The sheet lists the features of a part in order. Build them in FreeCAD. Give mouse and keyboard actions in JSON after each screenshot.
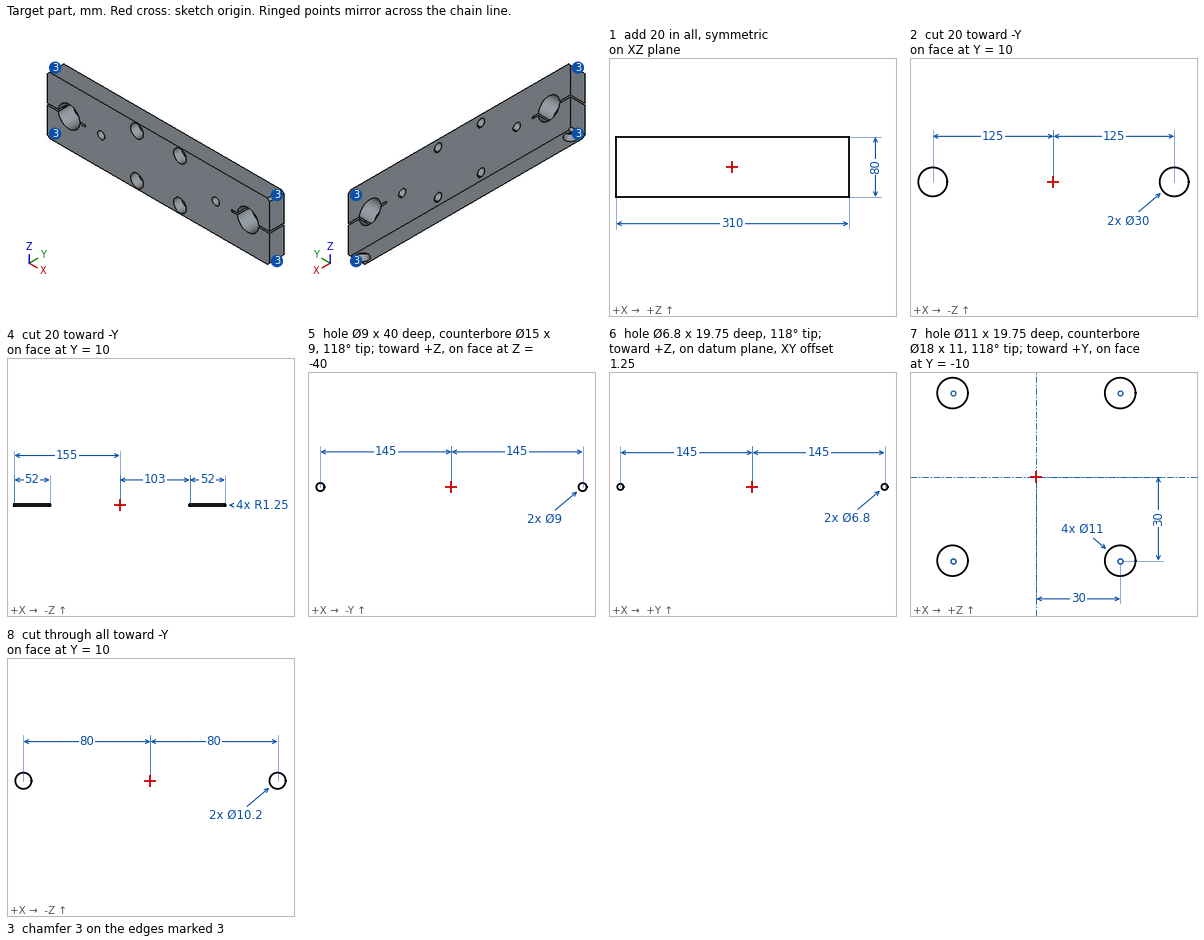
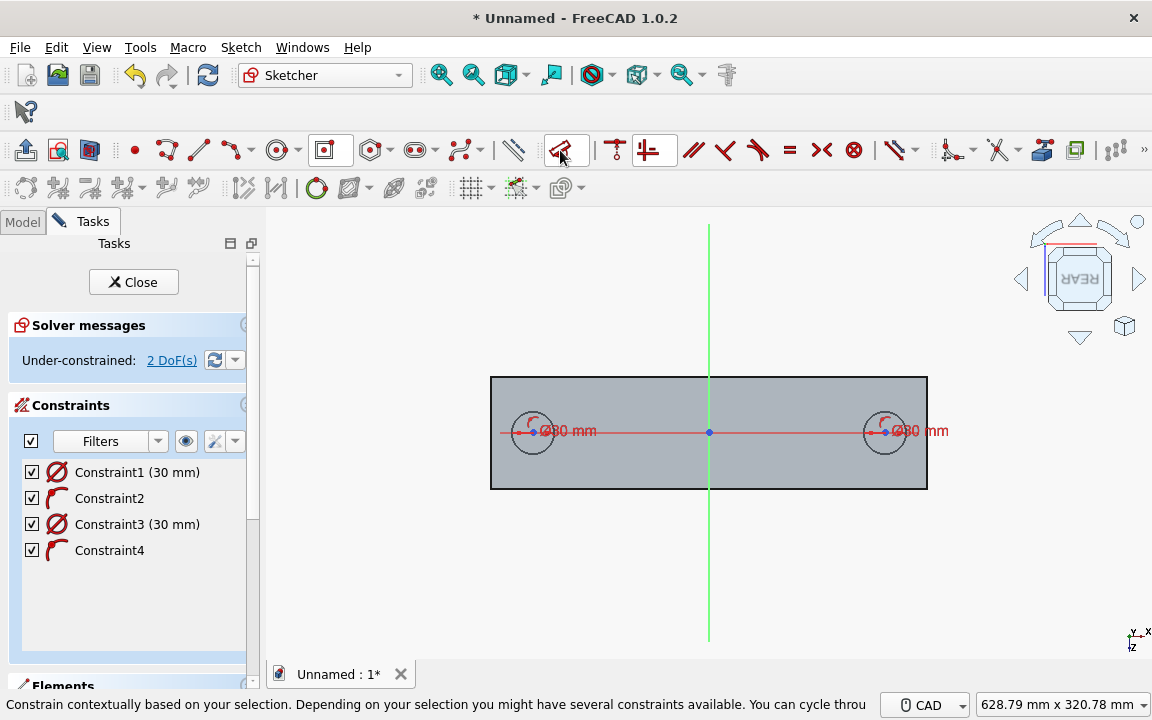
{"action": "left_click", "coordinate": [885, 433]}
{"action": "left_click", "coordinate": [797, 467]}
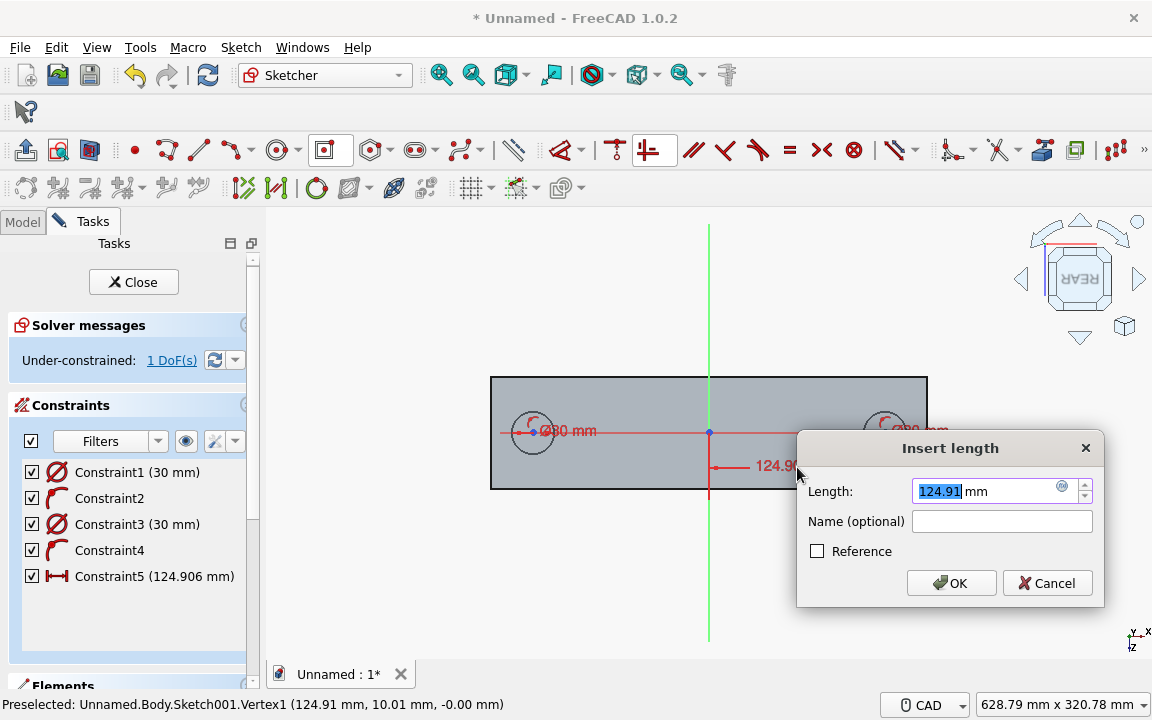
{"action": "type", "text": "125"}
{"action": "key", "text": "Return"}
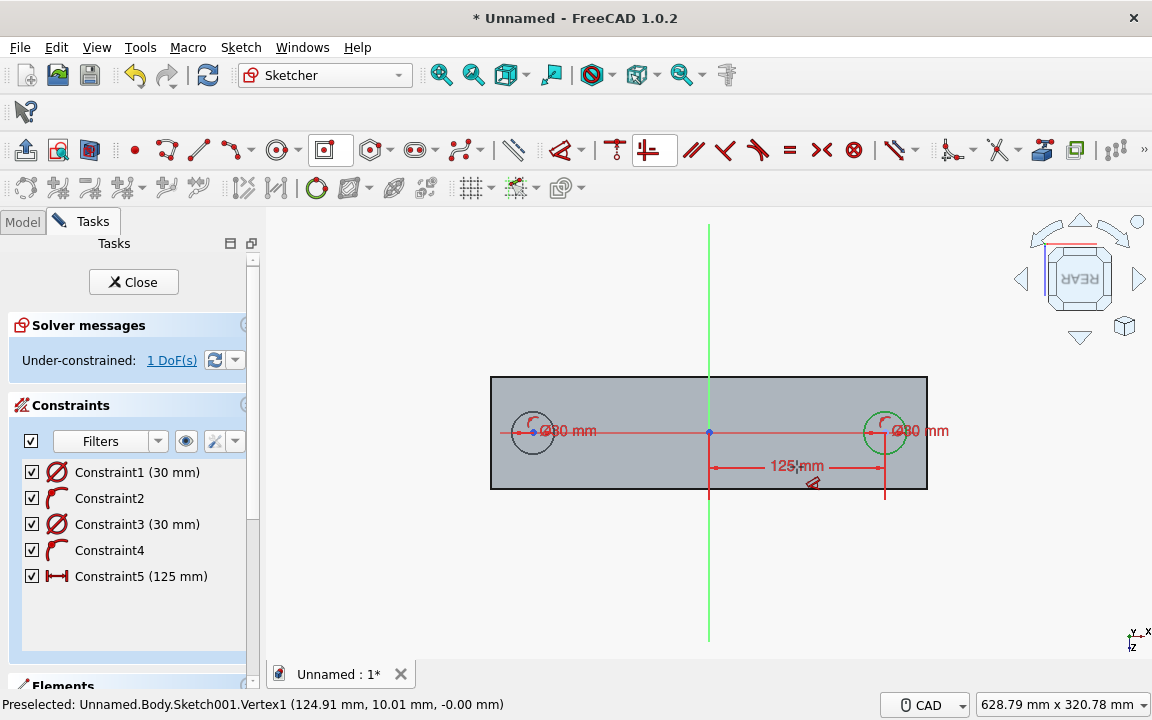
{"action": "left_click", "coordinate": [533, 433]}
{"action": "left_click", "coordinate": [621, 467]}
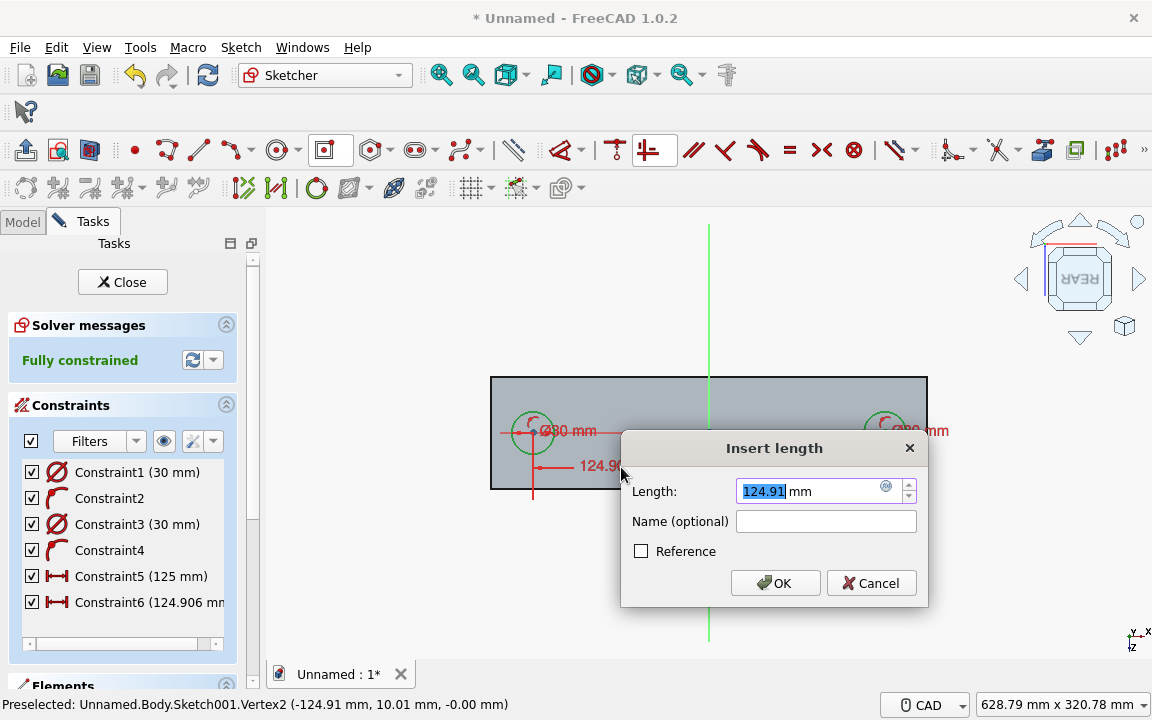
{"action": "type", "text": "125"}
{"action": "key", "text": "Return"}
{"action": "key", "text": "Escape"}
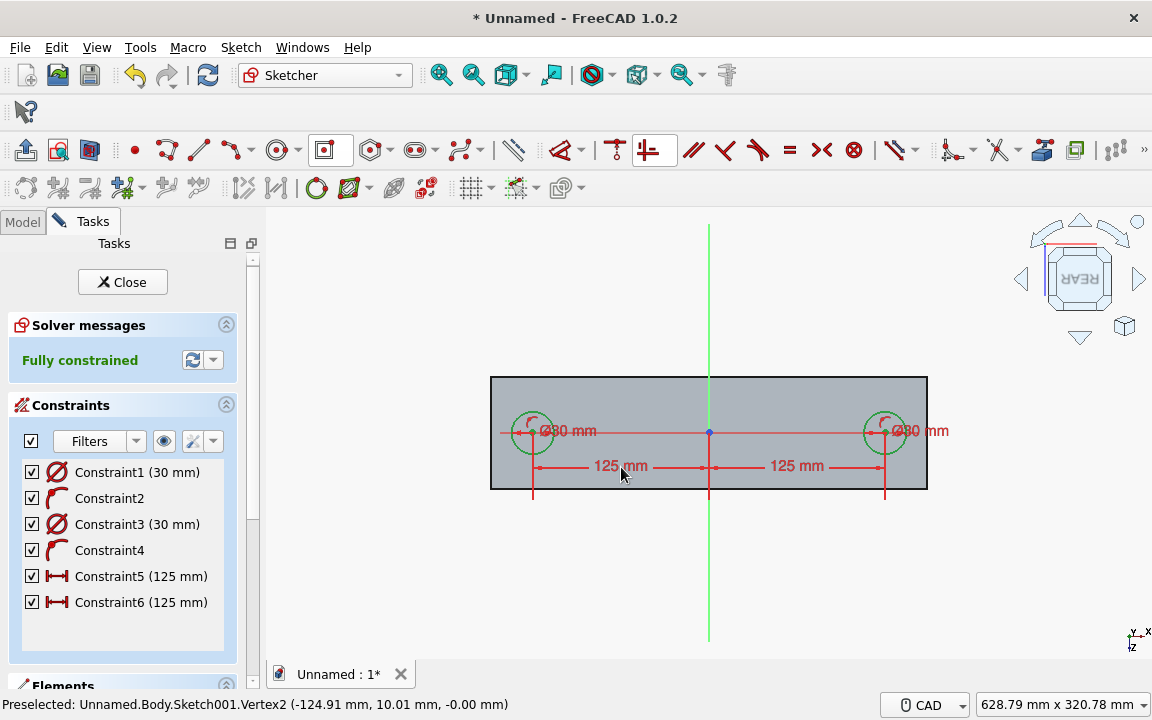
{"action": "left_click", "coordinate": [123, 282]}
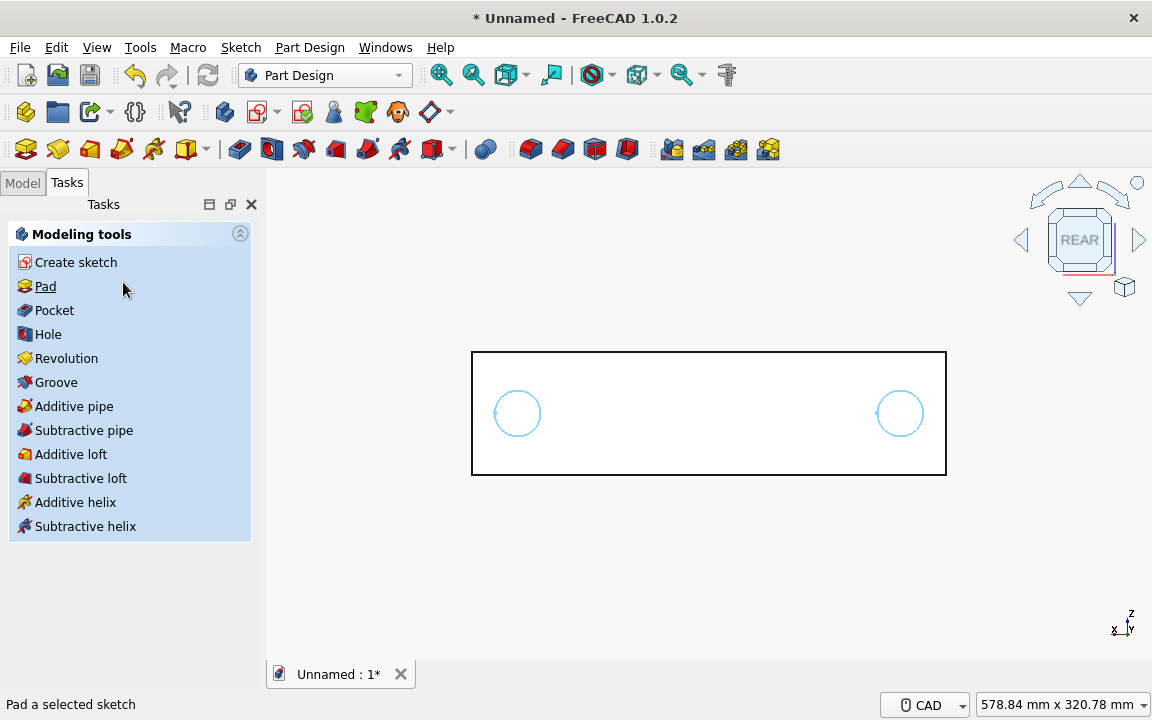
{"action": "left_click", "coordinate": [240, 150]}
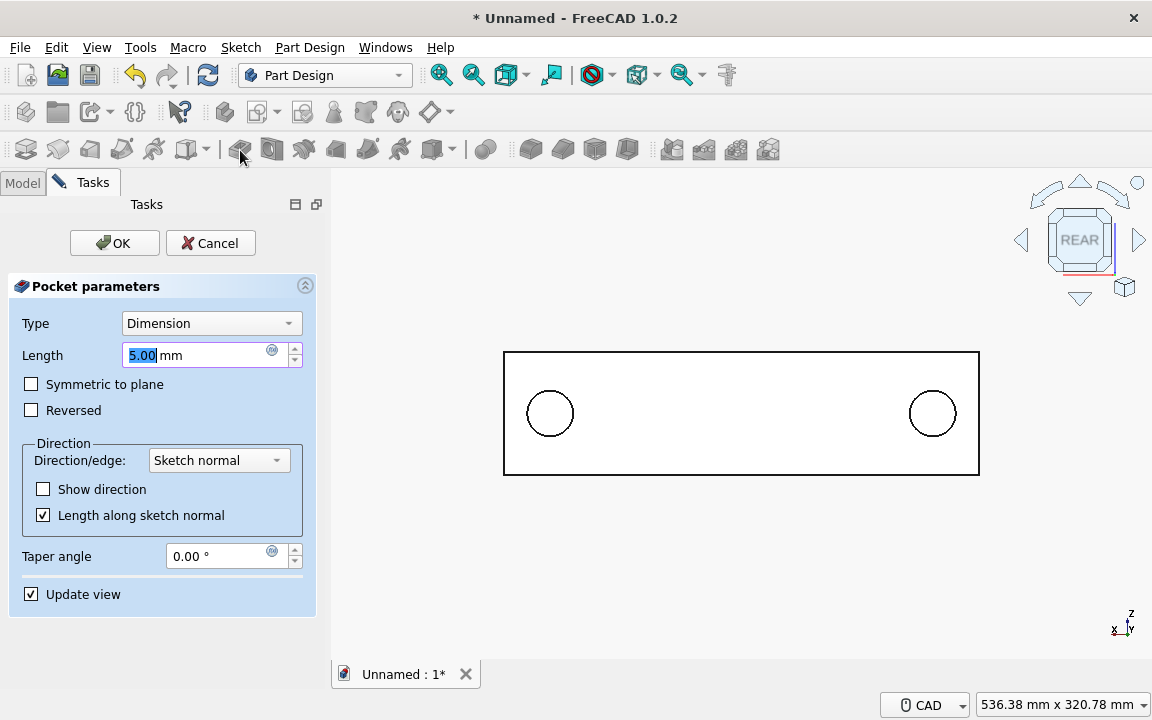
{"action": "type", "text": "20"}
{"action": "key", "text": "Tab"}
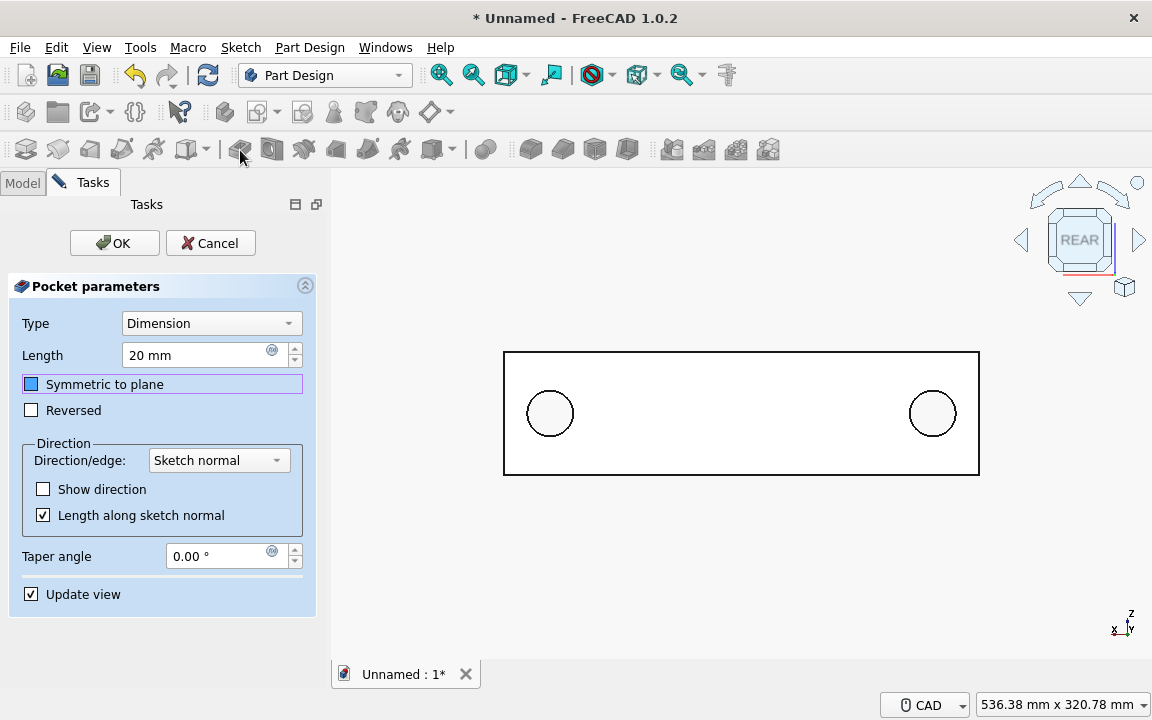
{"action": "left_click", "coordinate": [115, 243]}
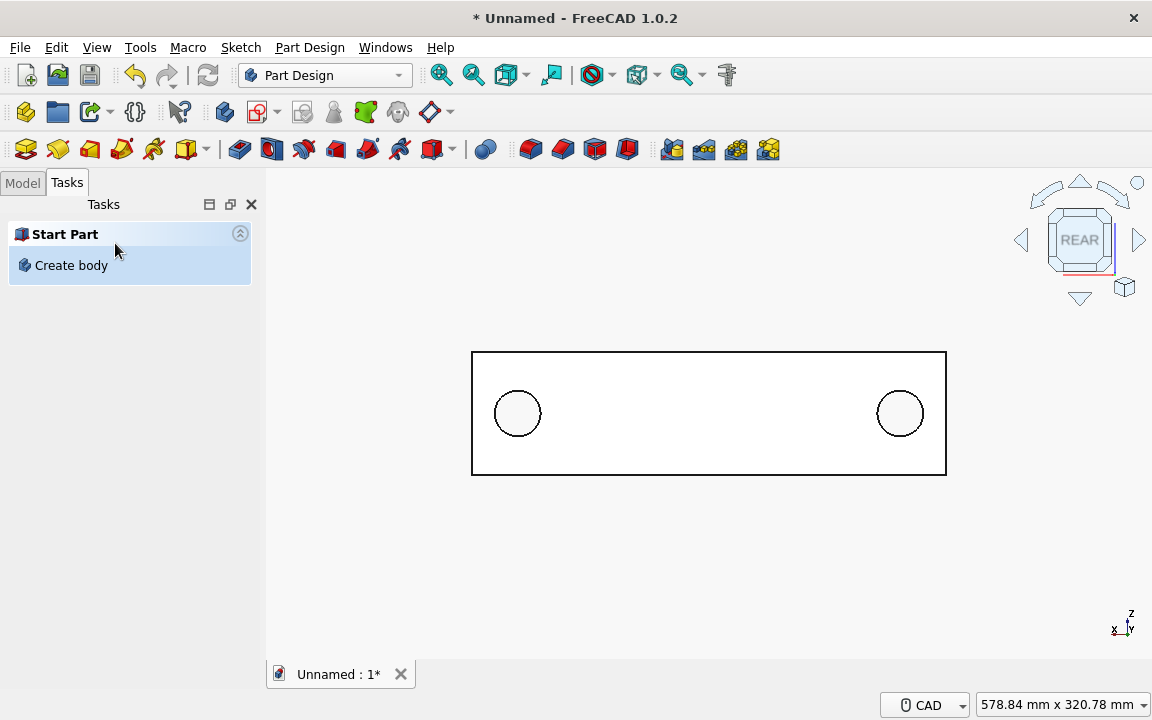
{"action": "key", "text": "0"}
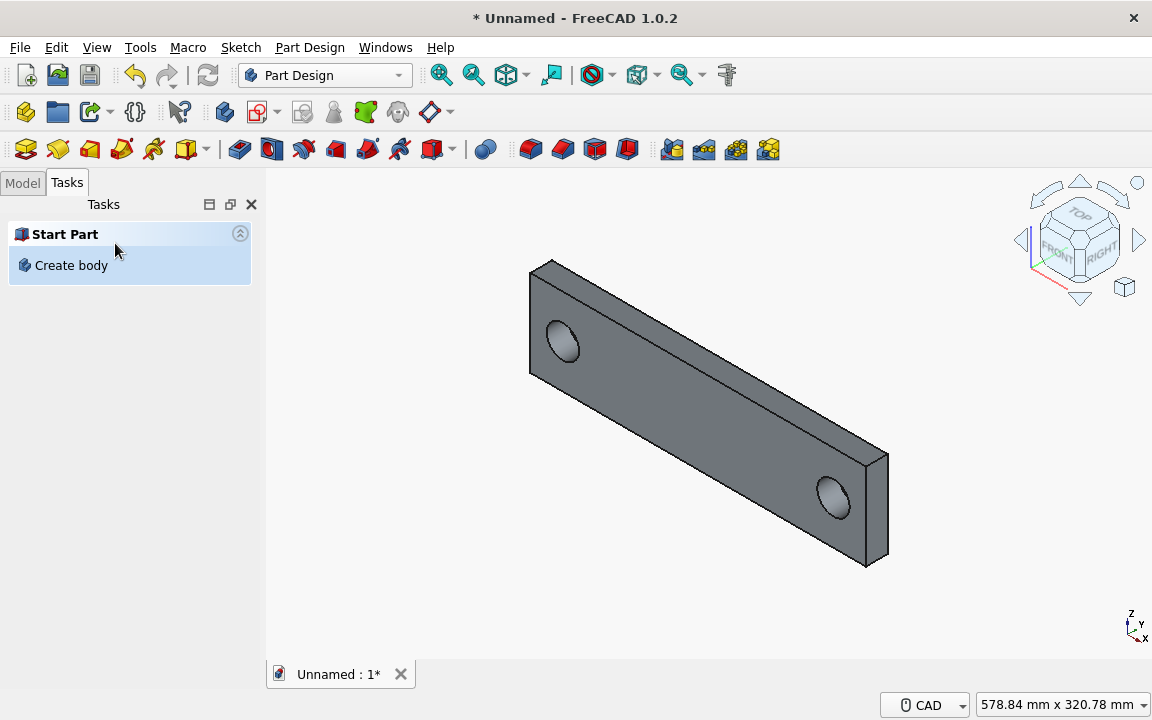
{"action": "left_click", "coordinate": [877, 459]}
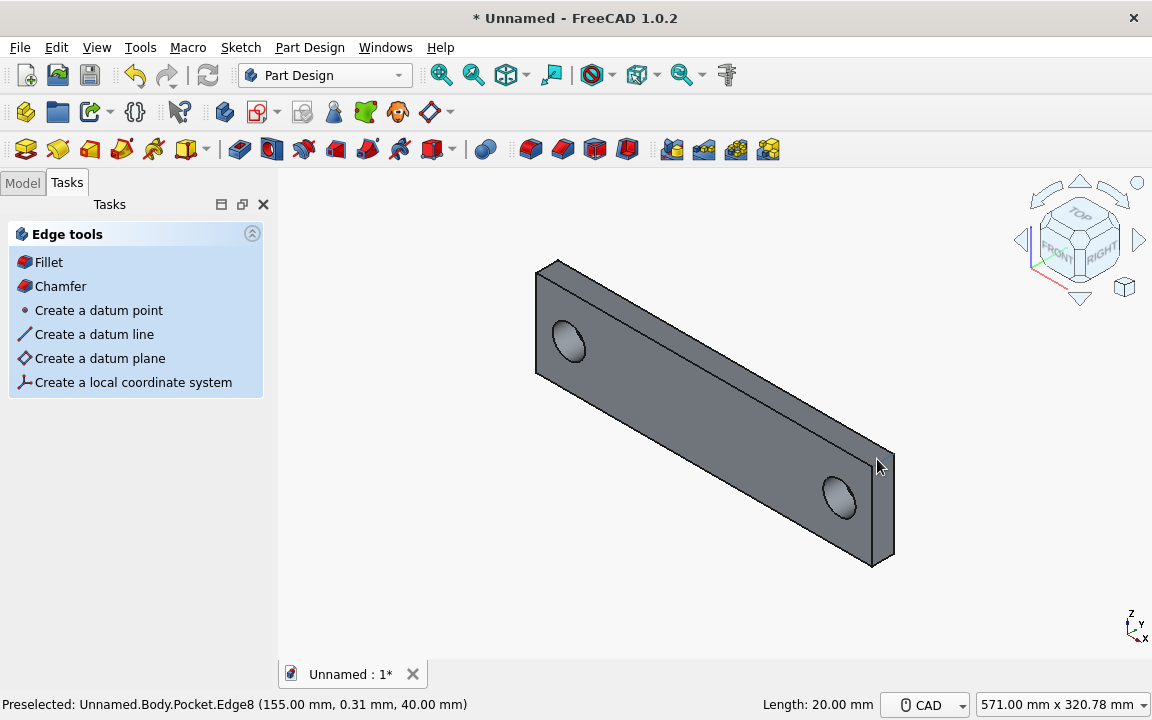
{"action": "key", "text": "2"}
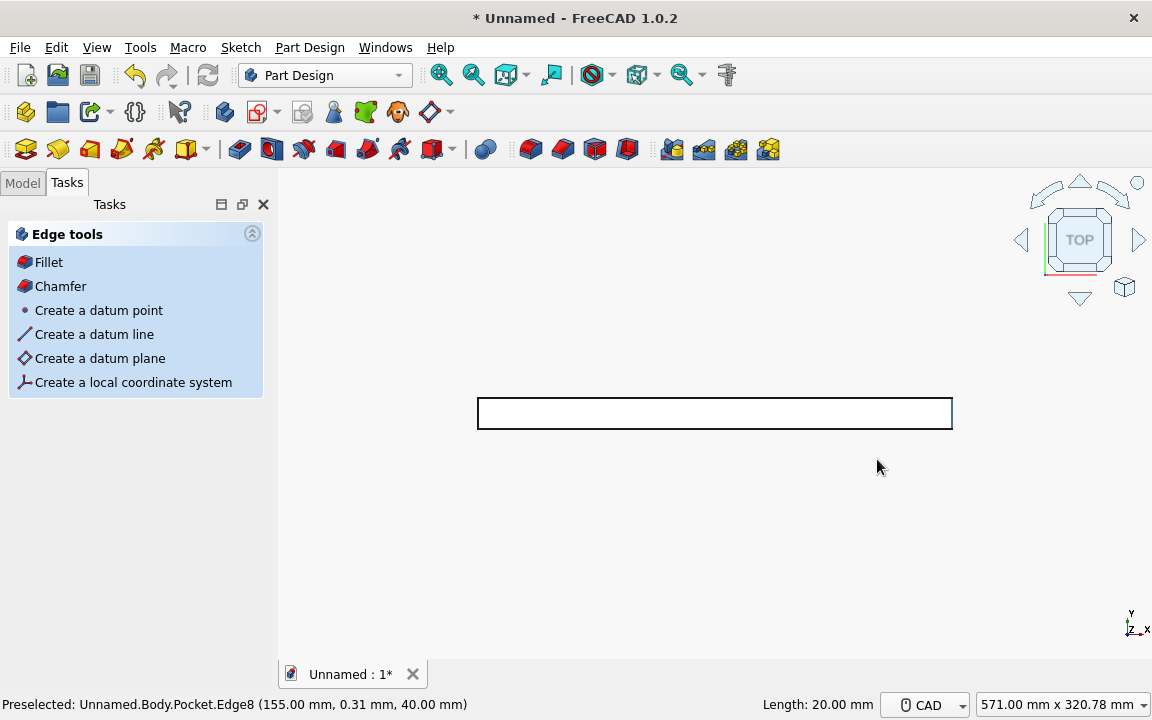
{"action": "left_click", "coordinate": [478, 412], "text": "ctrl"}